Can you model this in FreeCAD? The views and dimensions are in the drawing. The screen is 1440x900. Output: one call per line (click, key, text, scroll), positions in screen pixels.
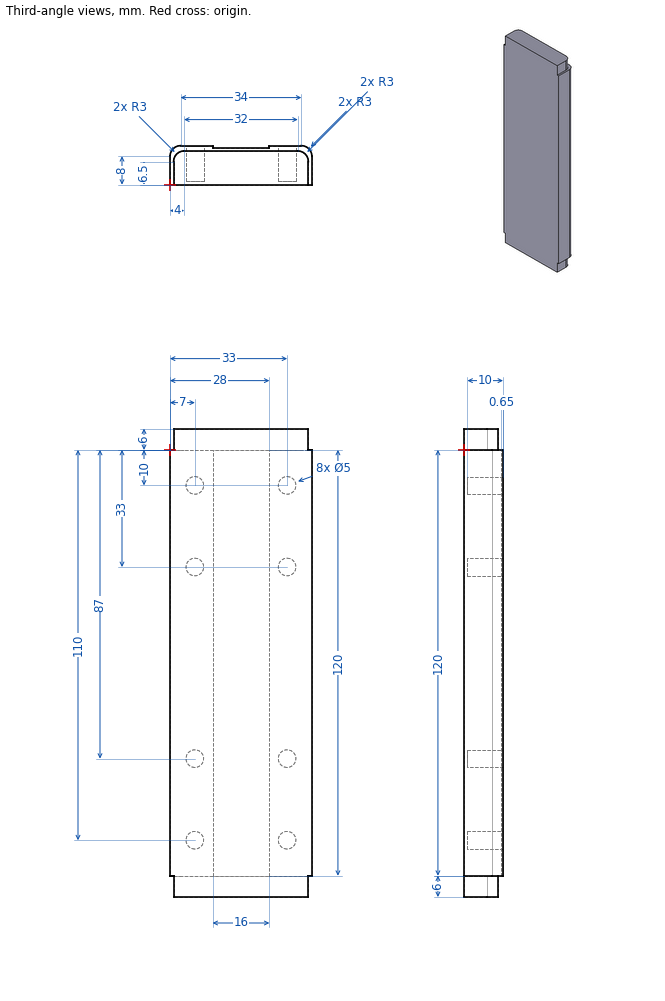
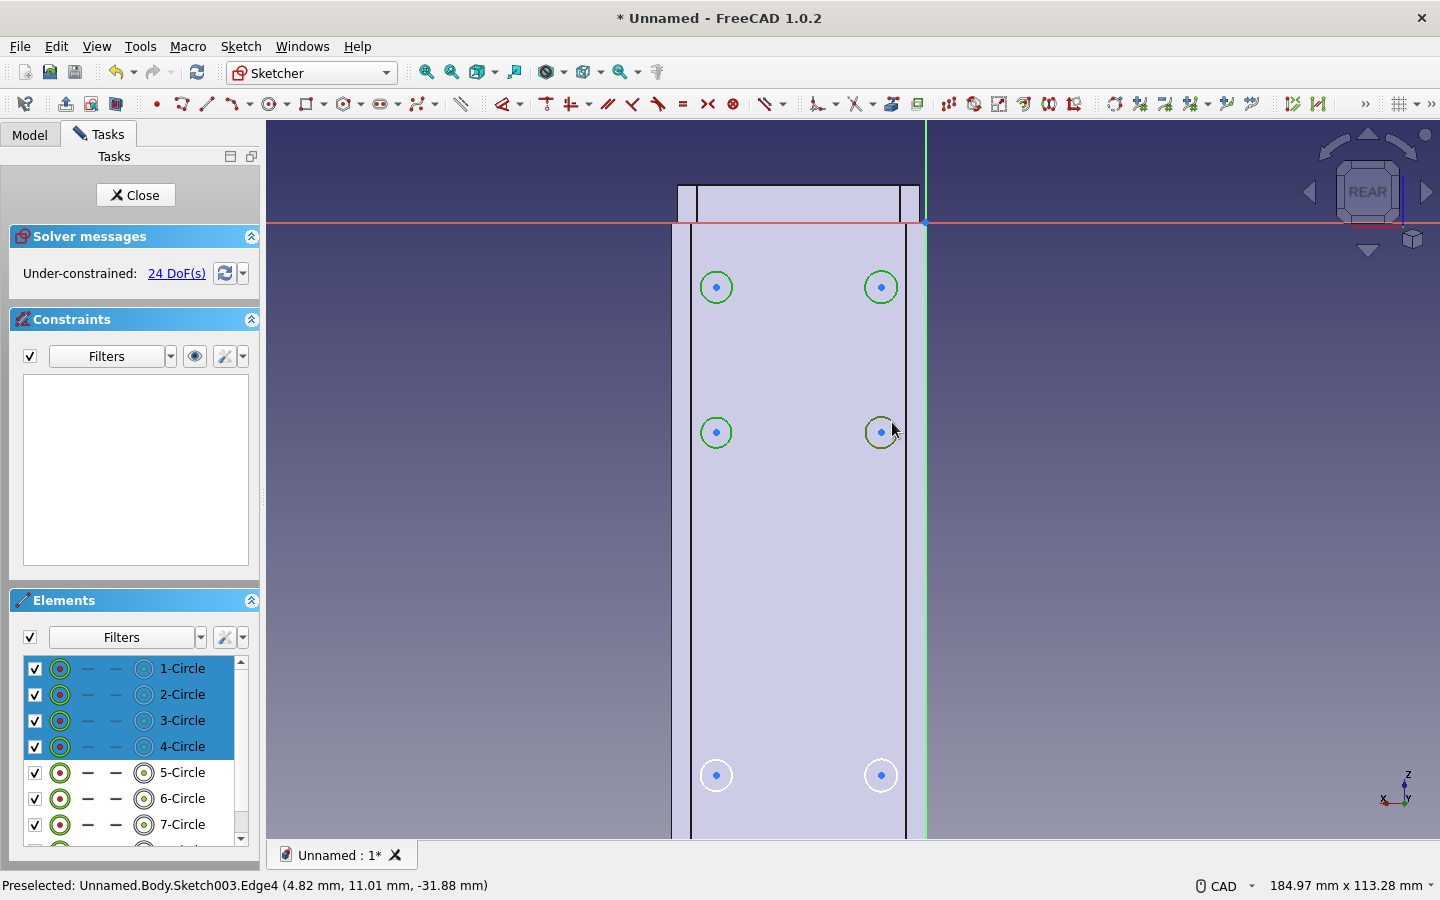
click(893, 764)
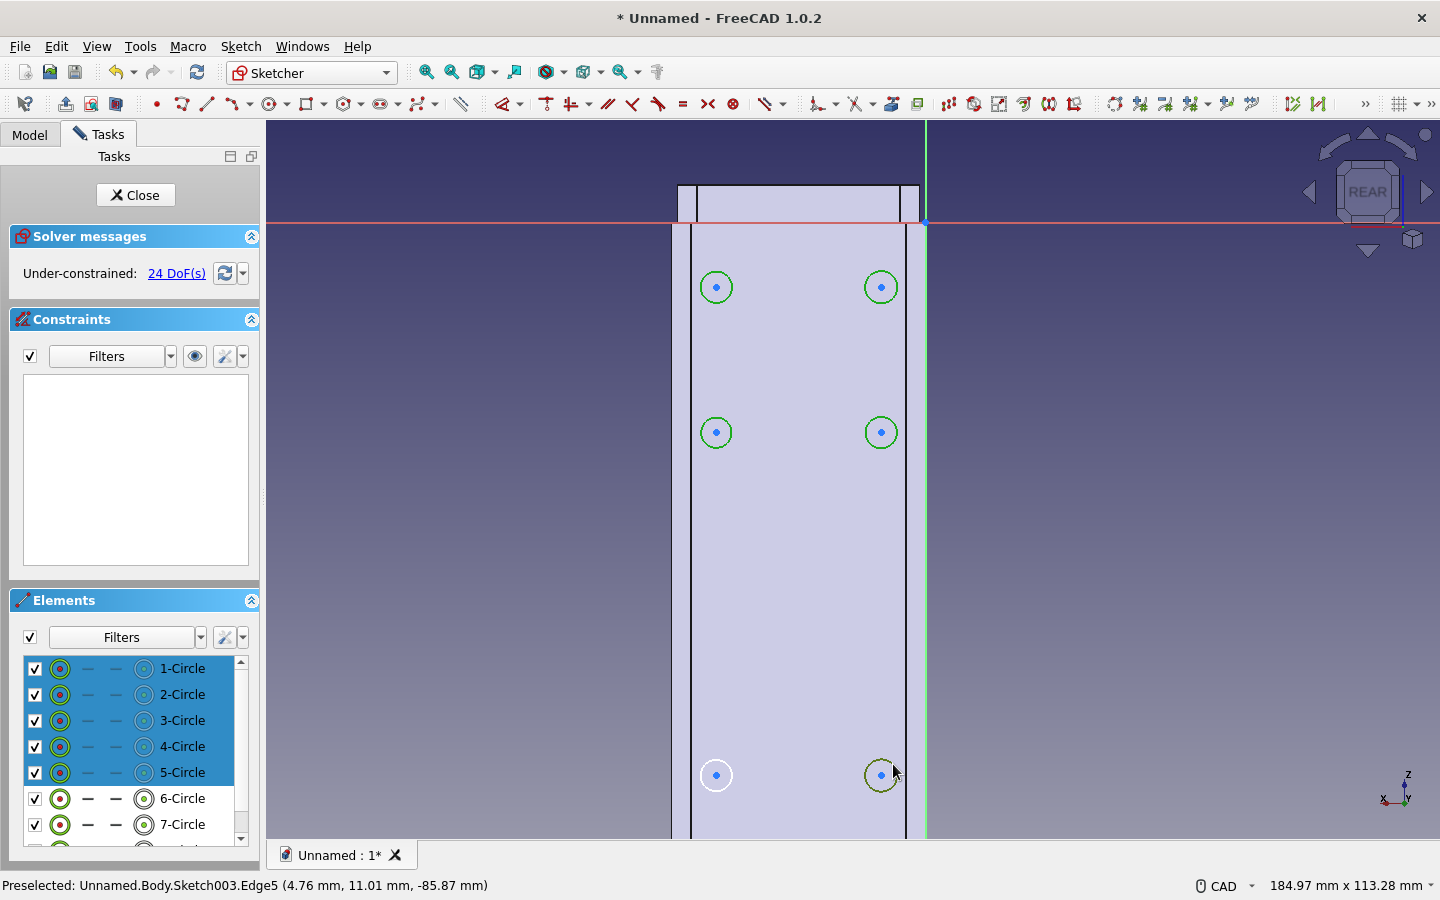
click(727, 764)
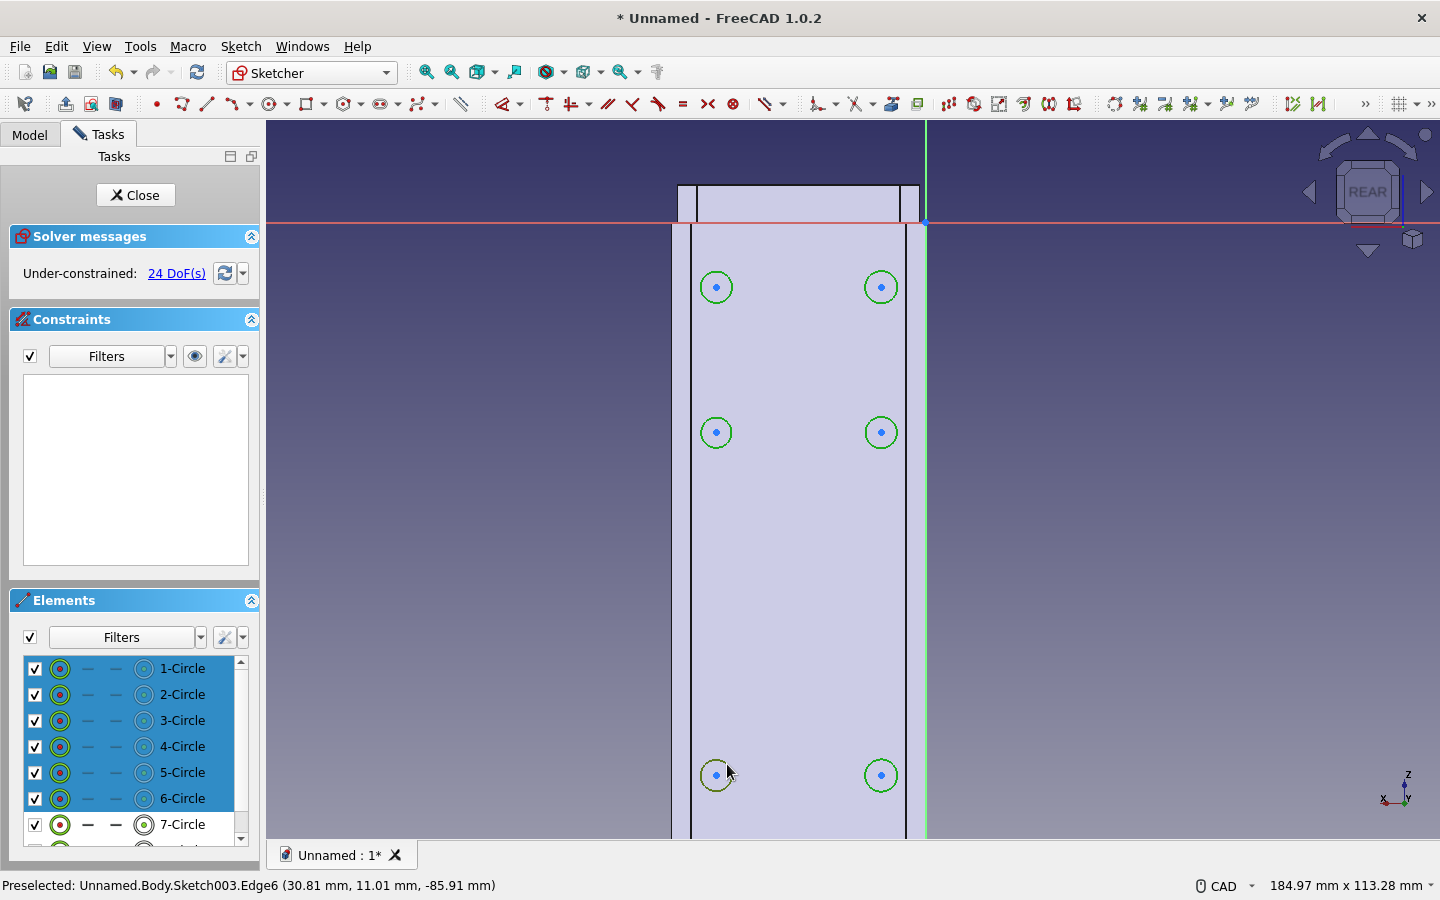
scroll(727, 276, down, 2)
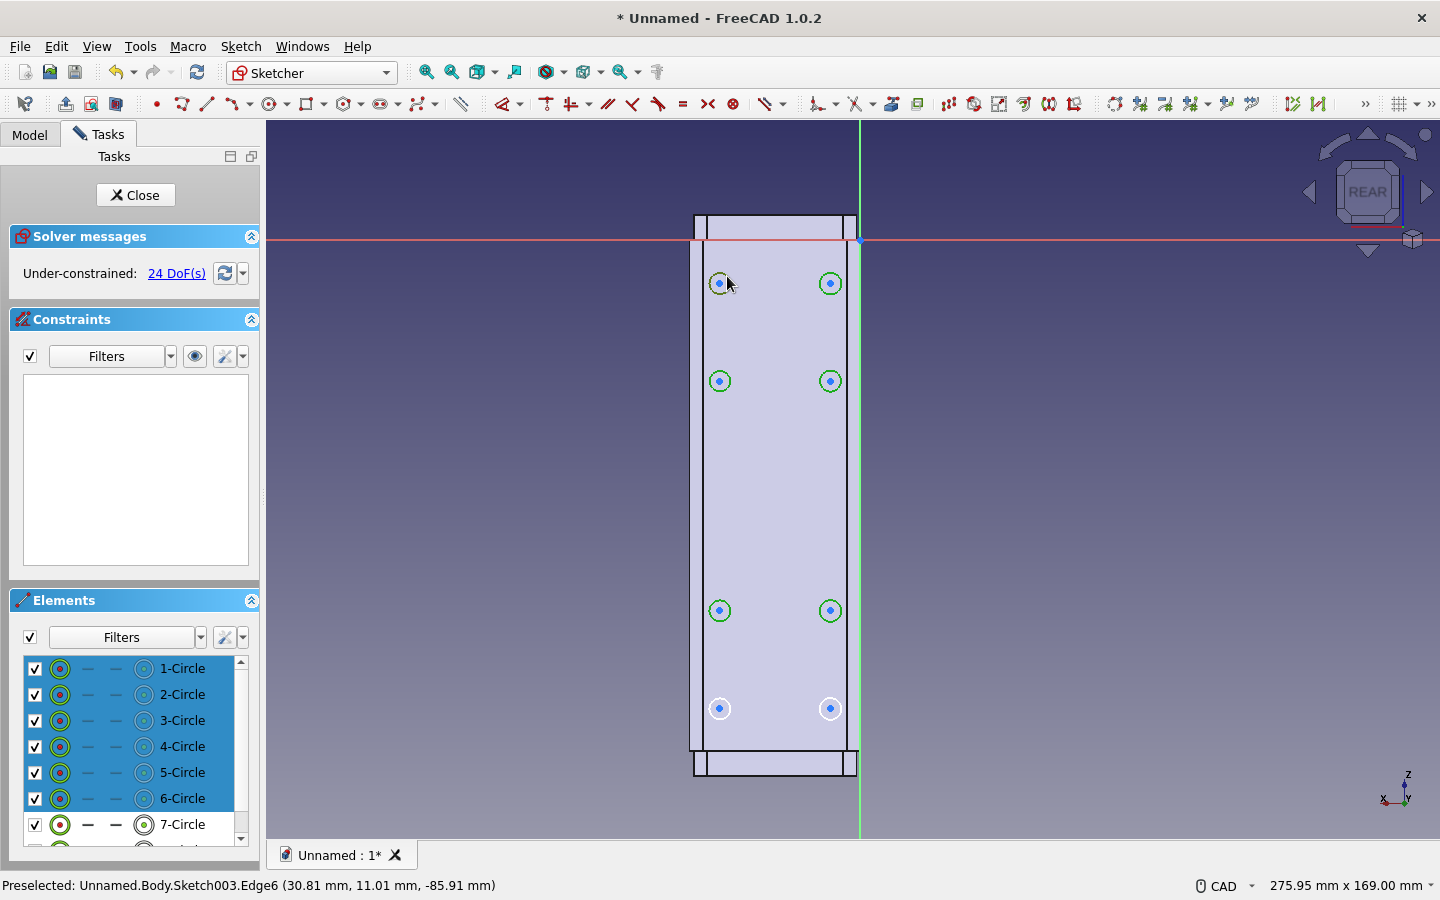
scroll(838, 701, up, 2)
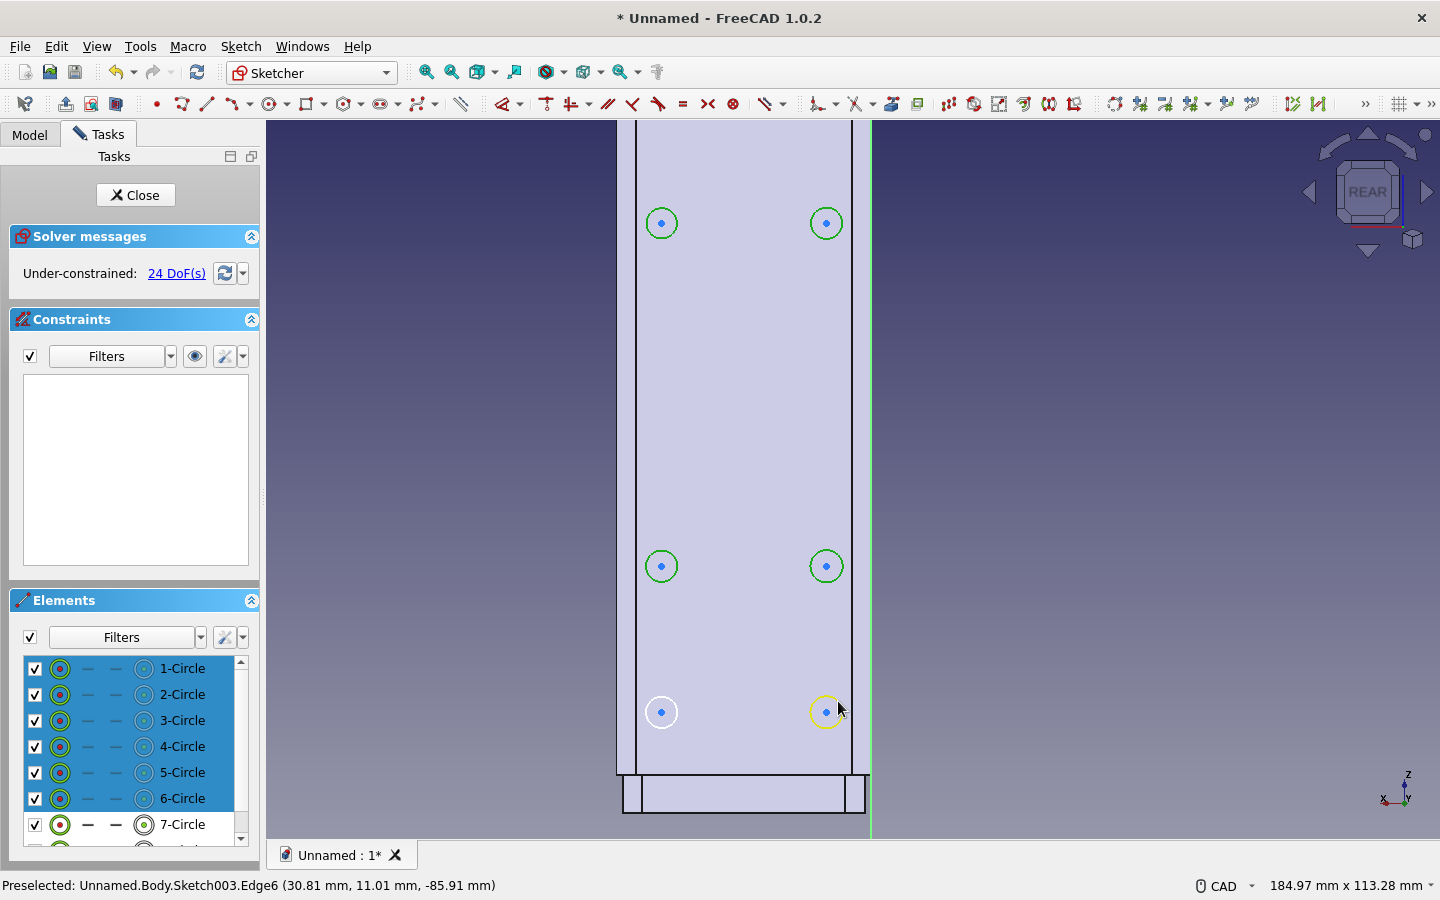
click(838, 701)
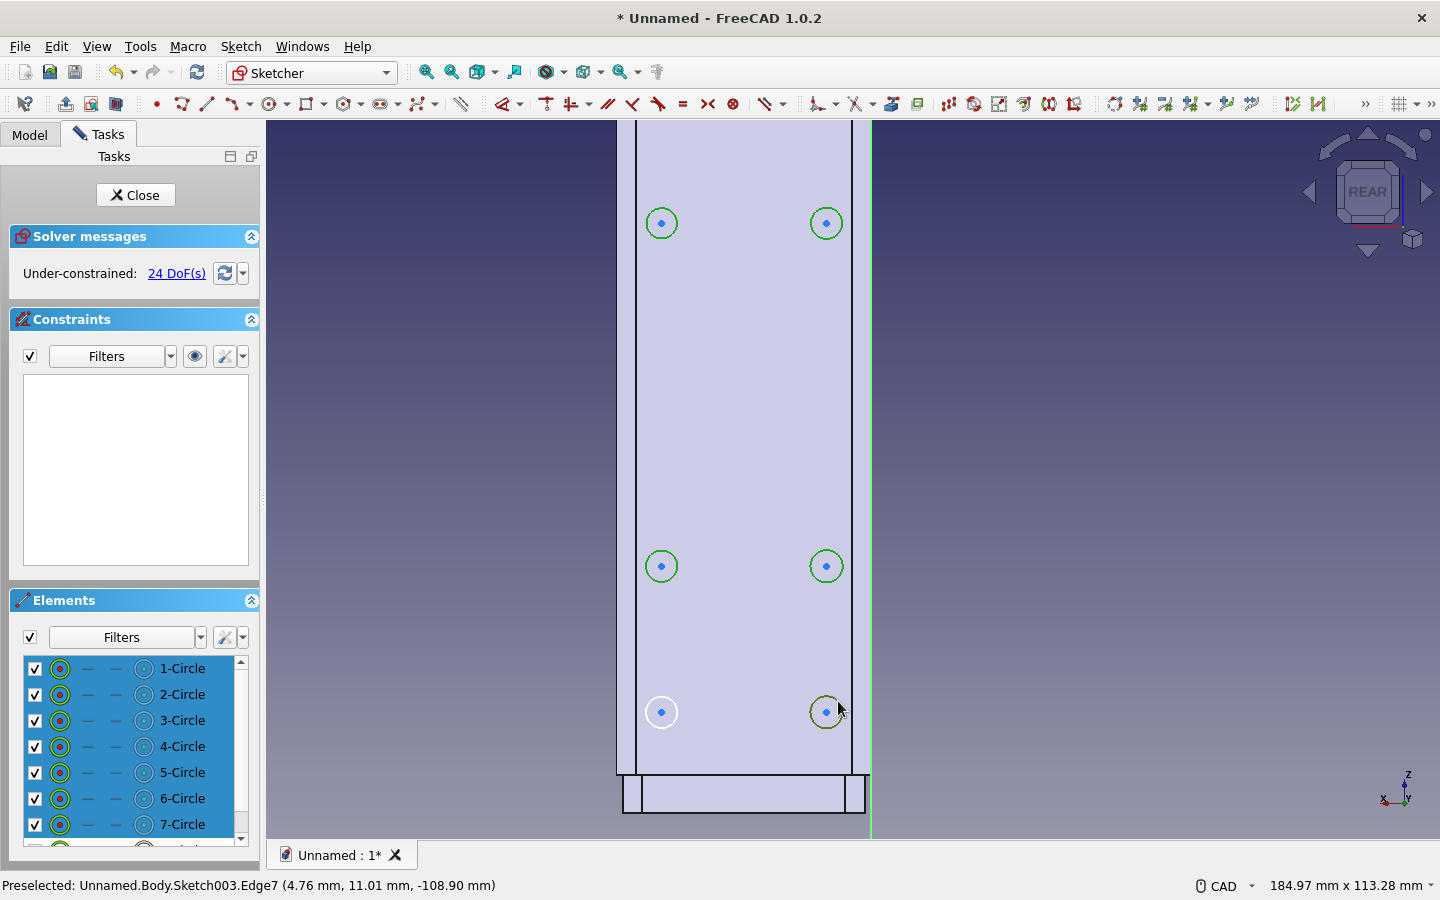
click(673, 701)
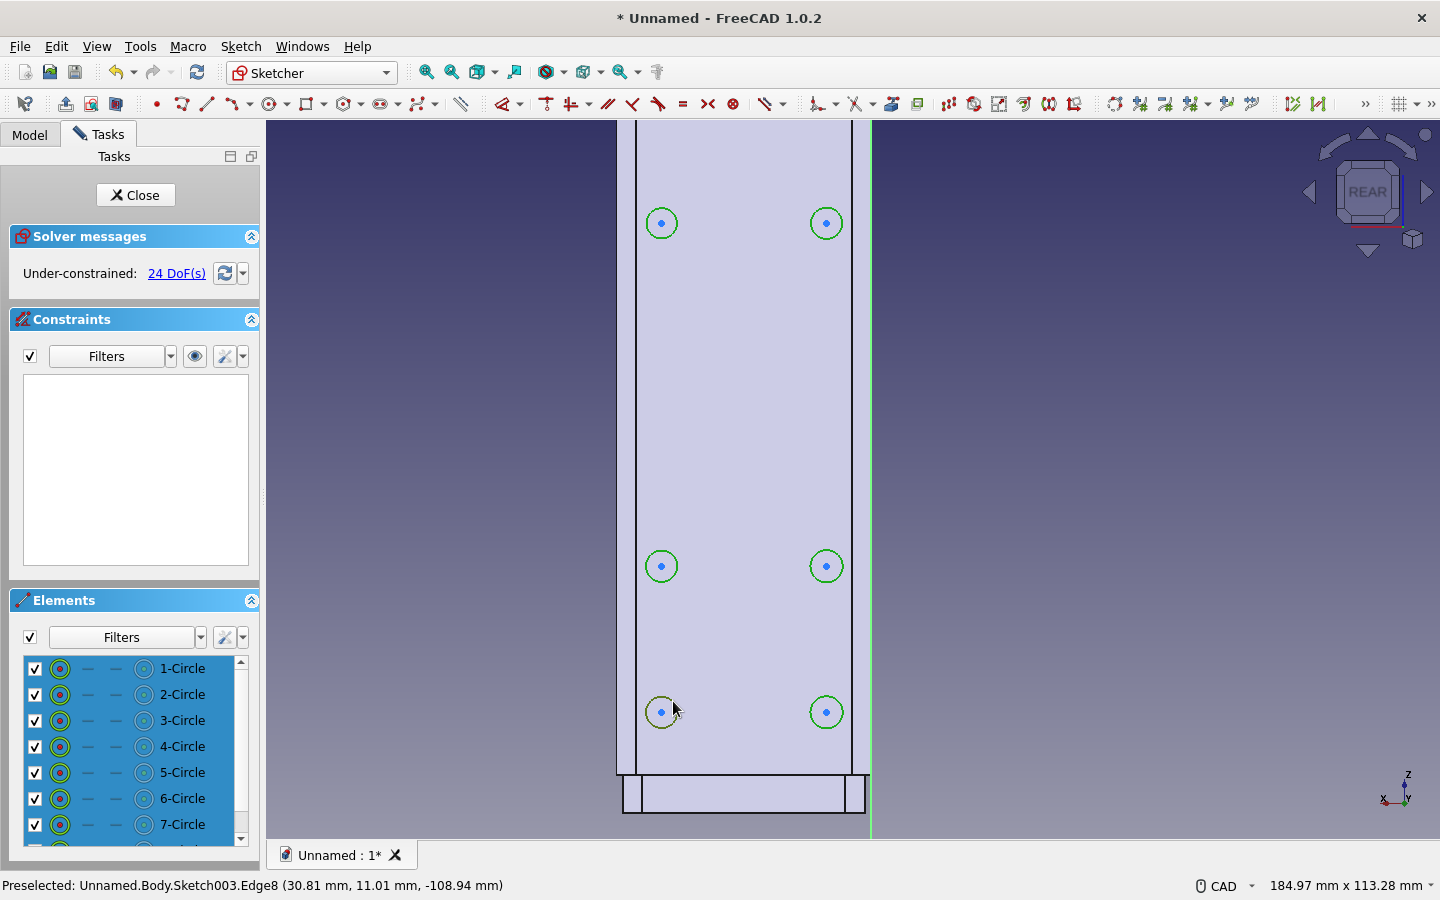
click(683, 104)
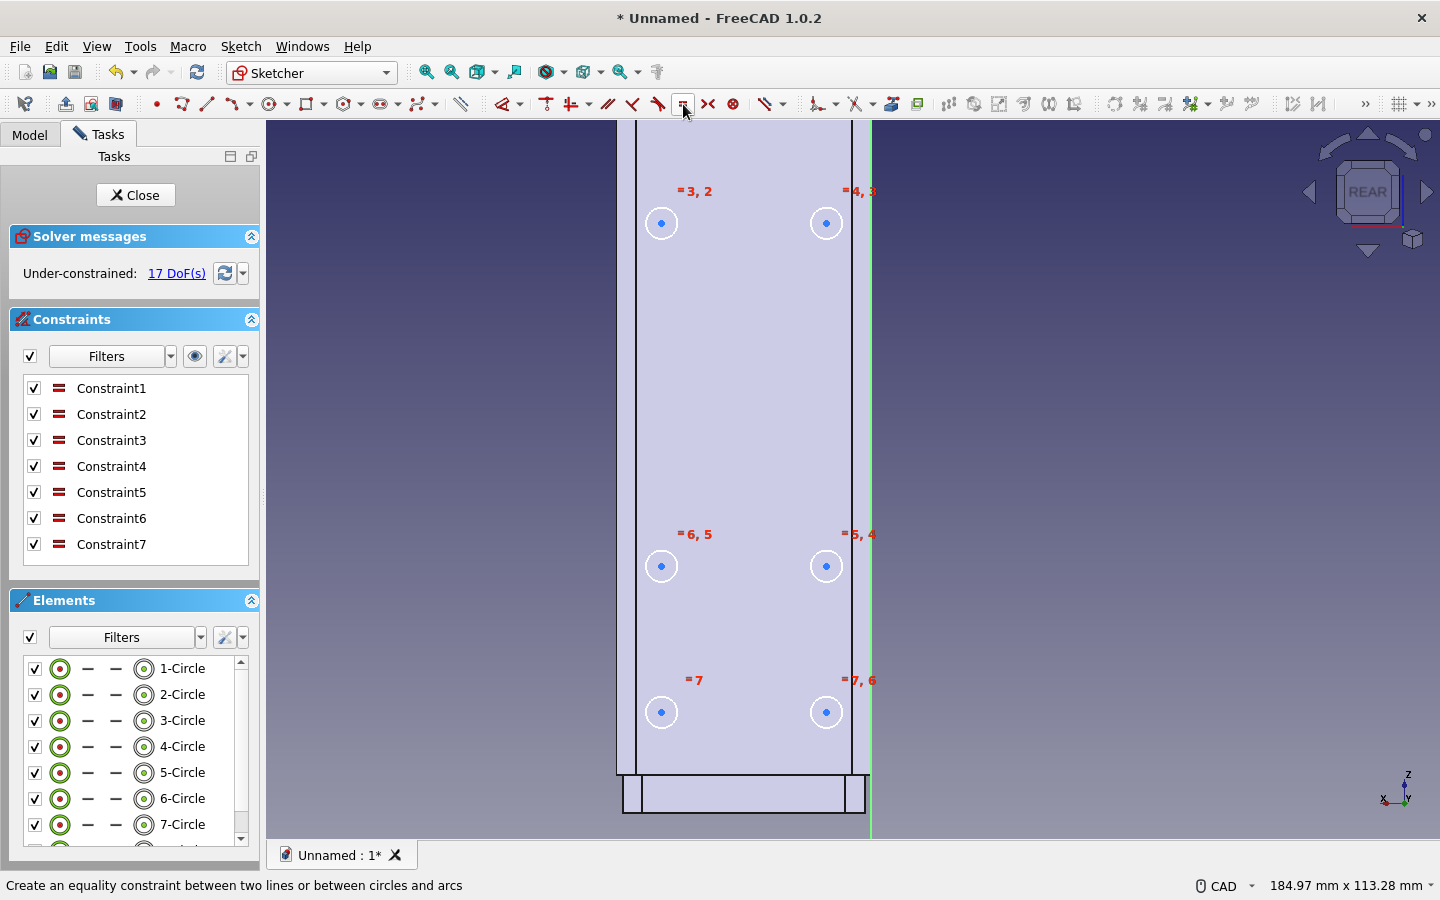
scroll(838, 701, down, 2)